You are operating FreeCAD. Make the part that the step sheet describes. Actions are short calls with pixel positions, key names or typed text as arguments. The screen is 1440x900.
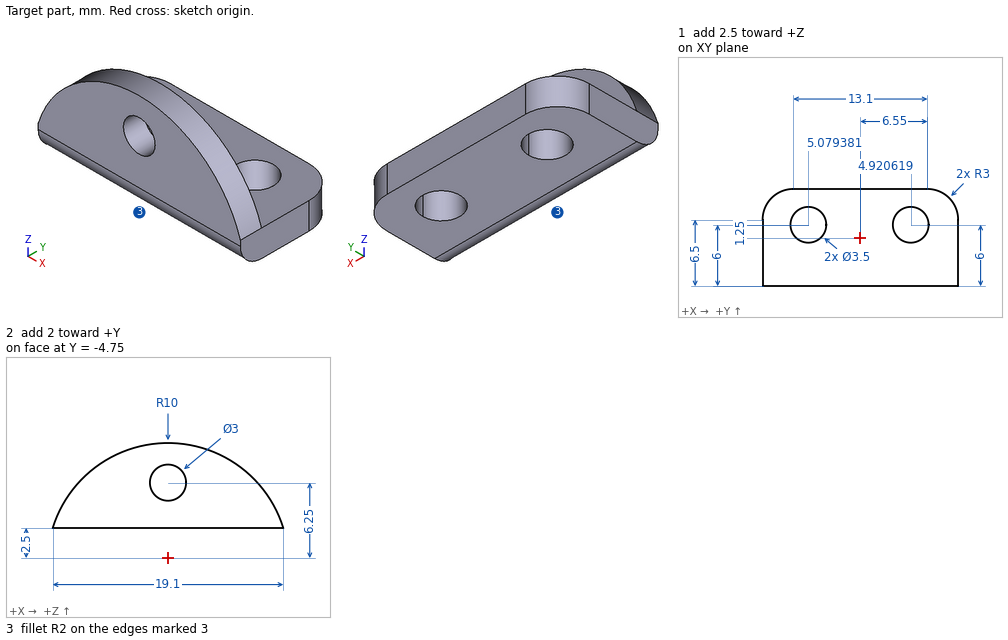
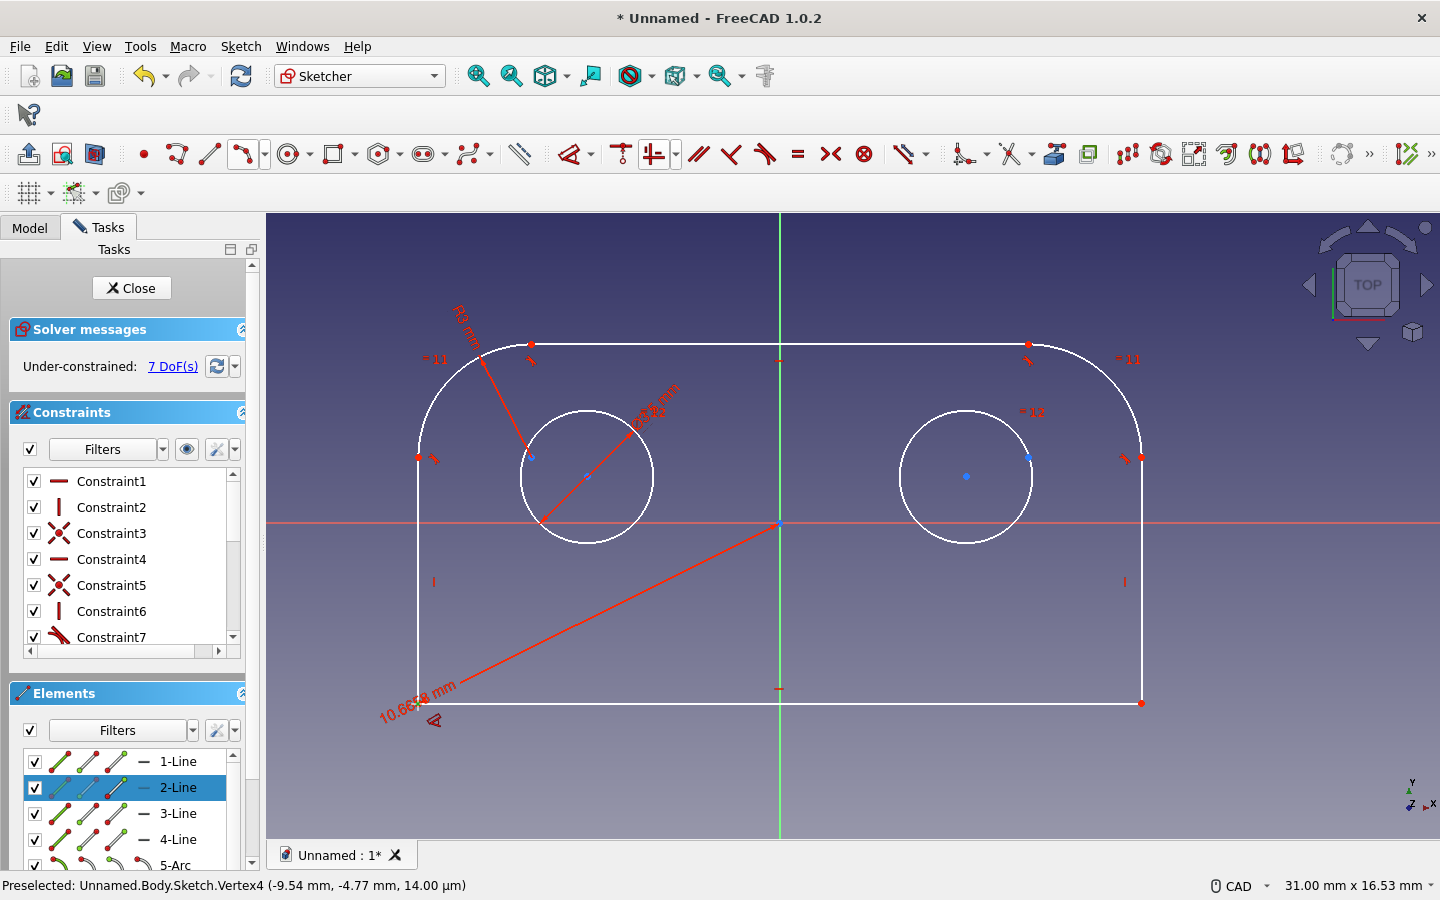
click(587, 477)
click(384, 590)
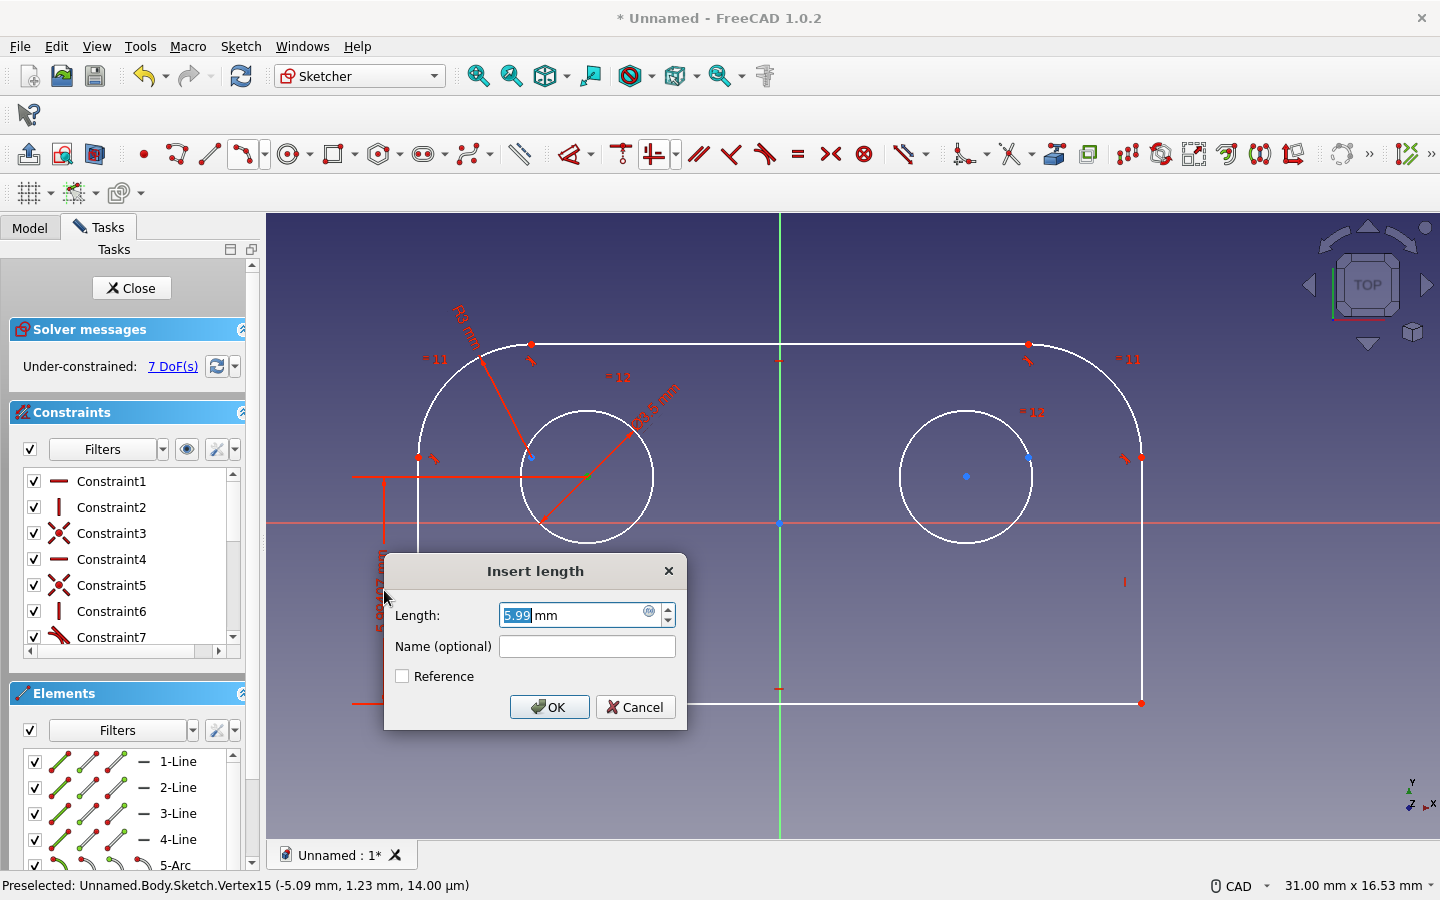
text(6)
key(Return)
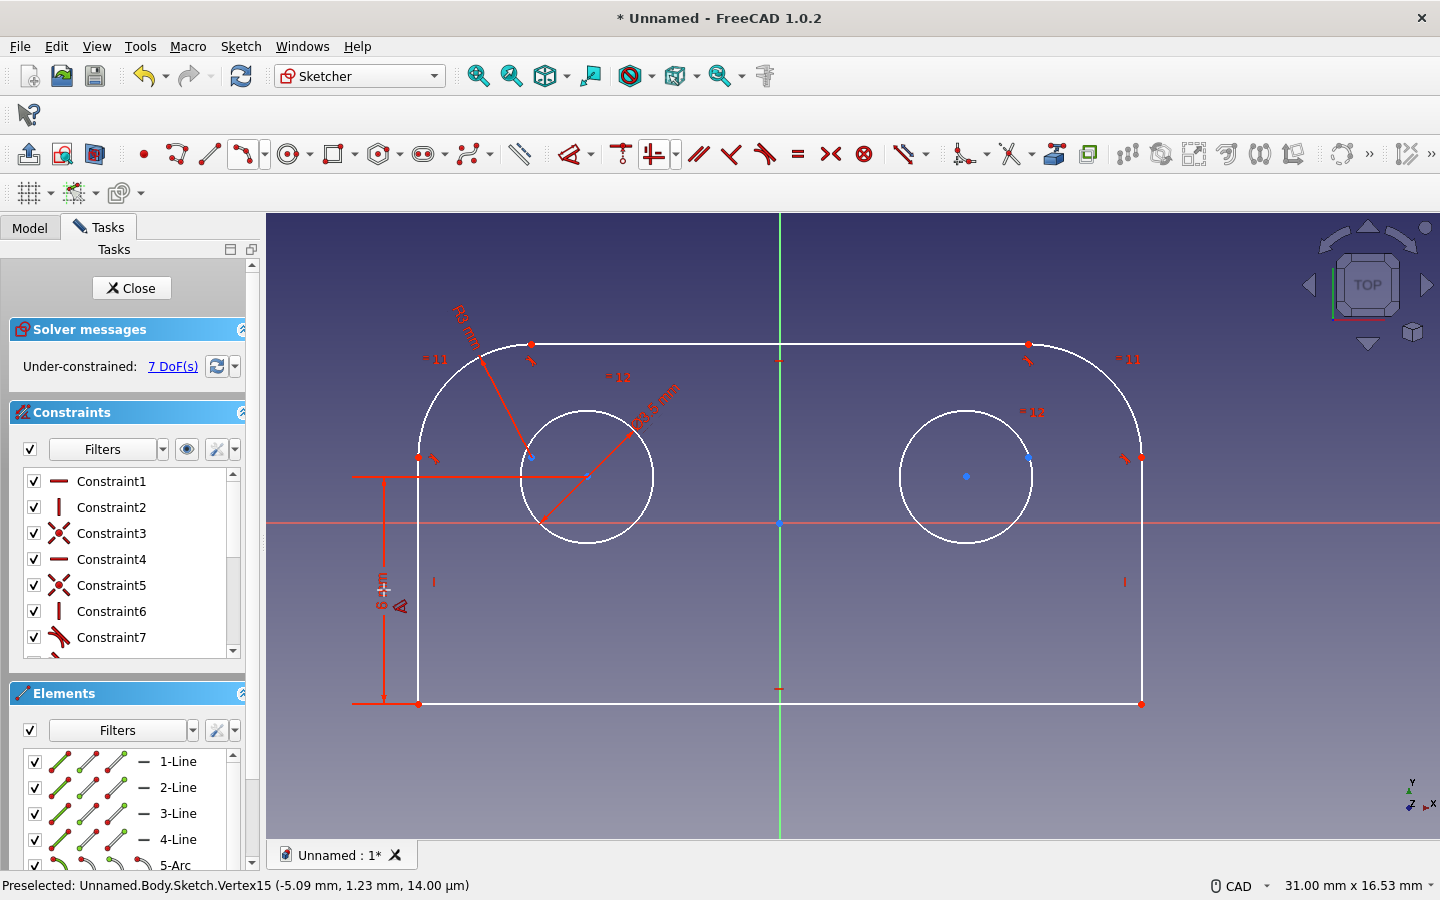
click(1142, 704)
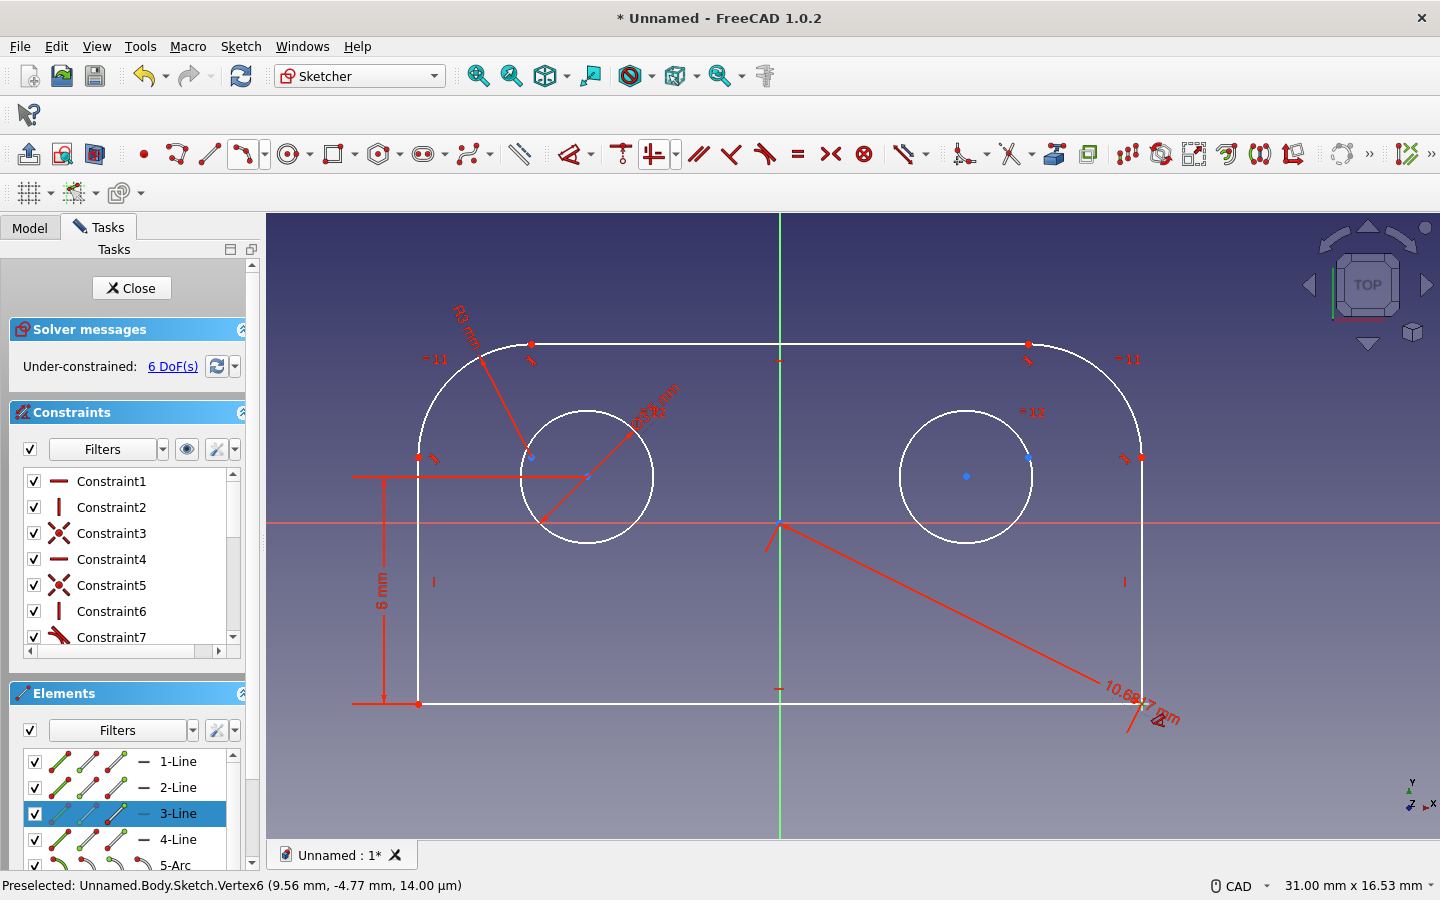
click(966, 477)
click(1176, 591)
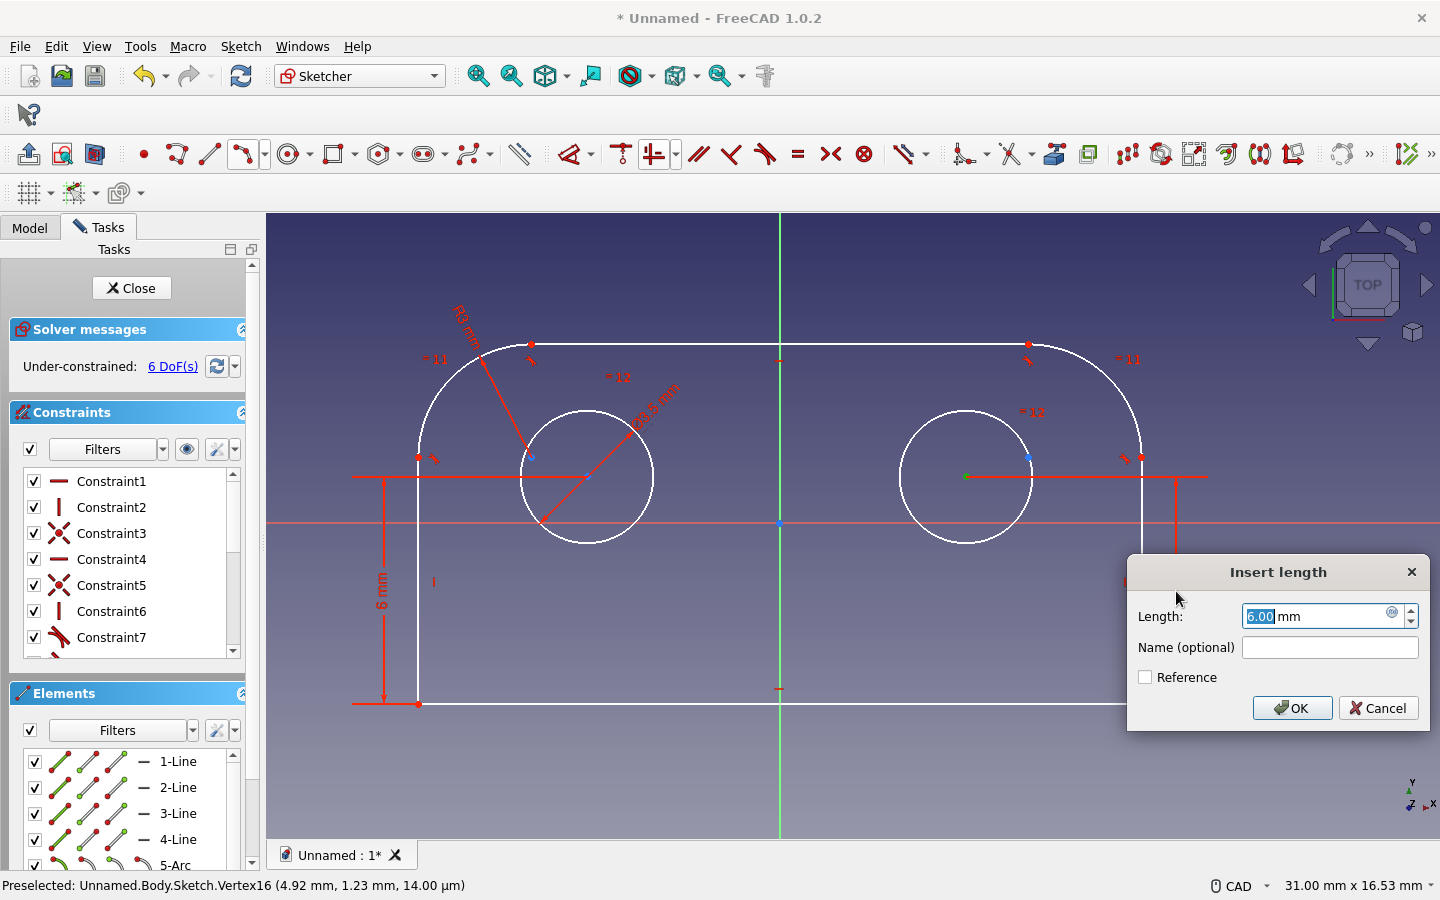
text(6)
key(Return)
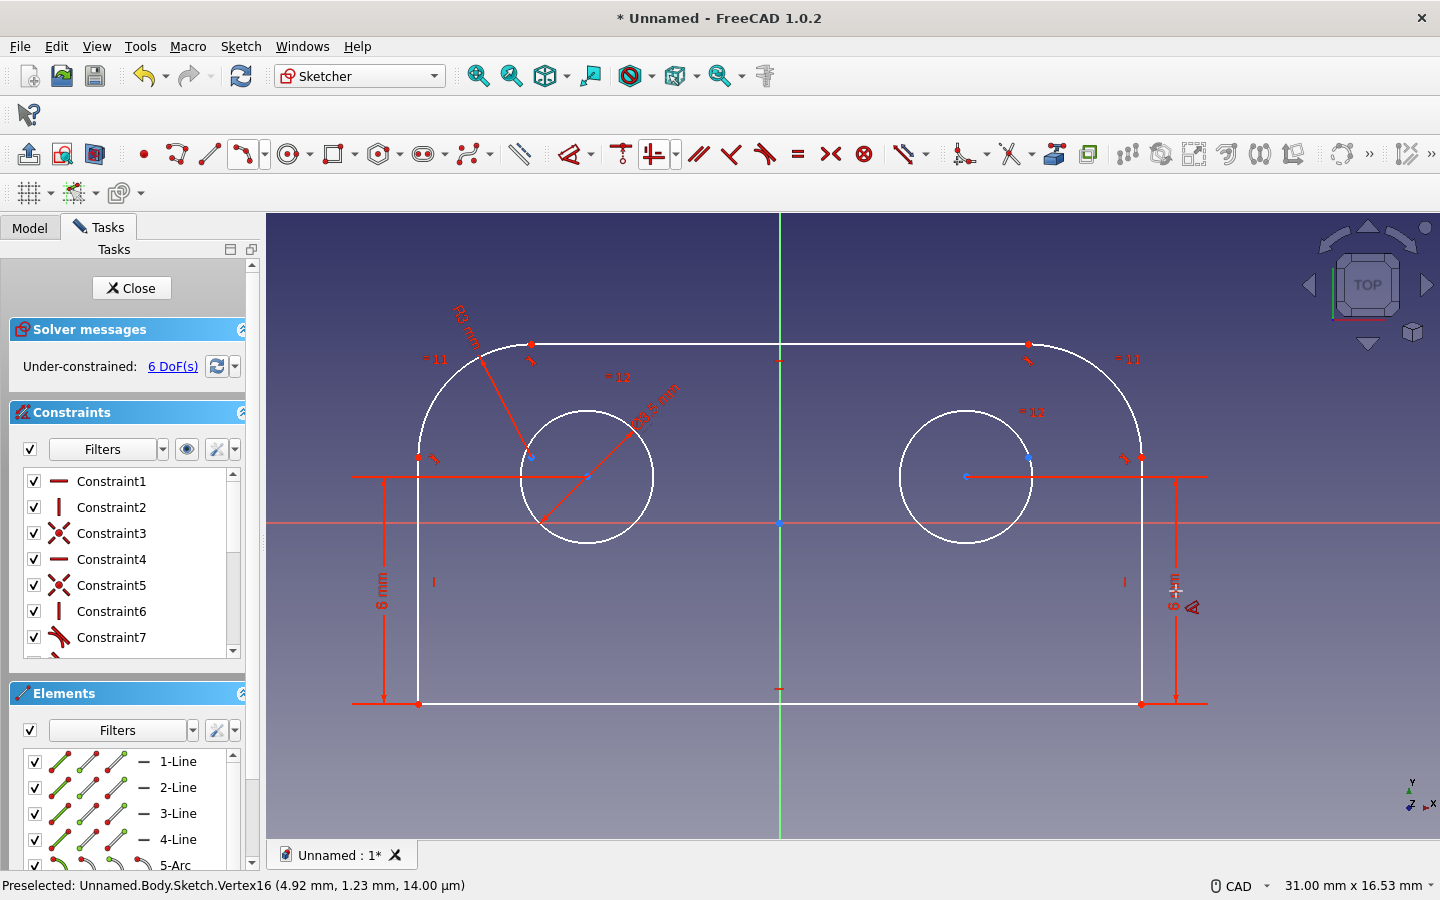
click(418, 630)
click(384, 638)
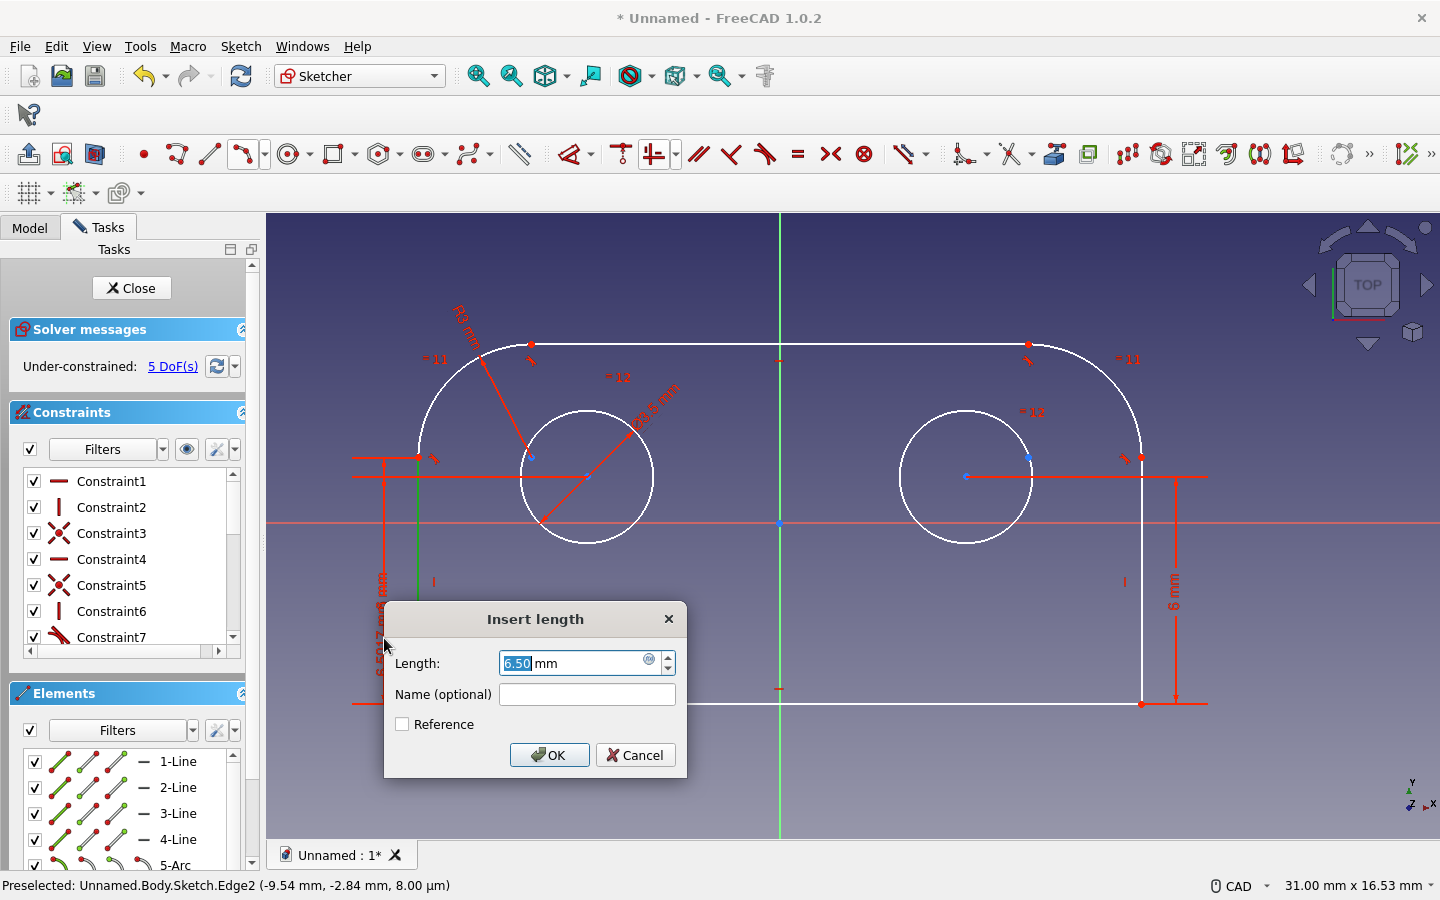
text(6.5)
key(Return)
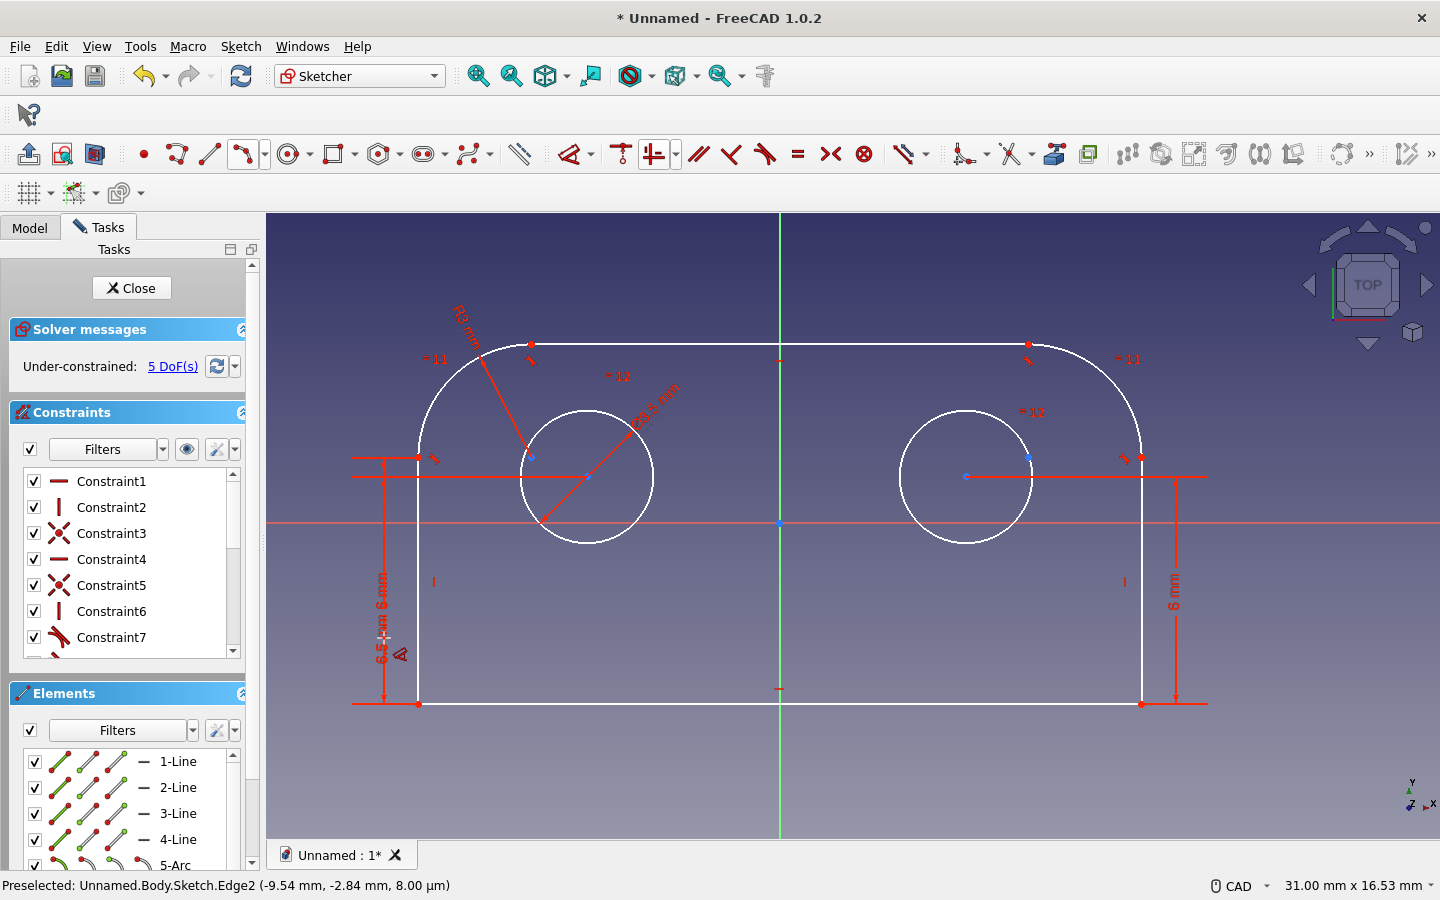
click(879, 344)
click(666, 310)